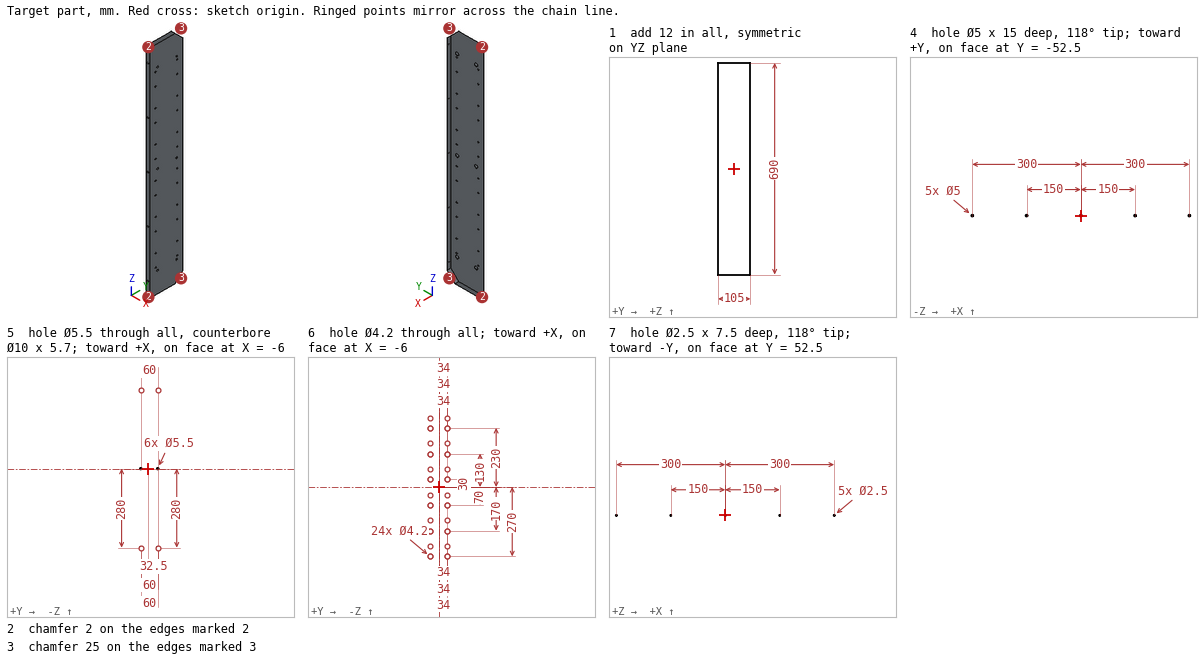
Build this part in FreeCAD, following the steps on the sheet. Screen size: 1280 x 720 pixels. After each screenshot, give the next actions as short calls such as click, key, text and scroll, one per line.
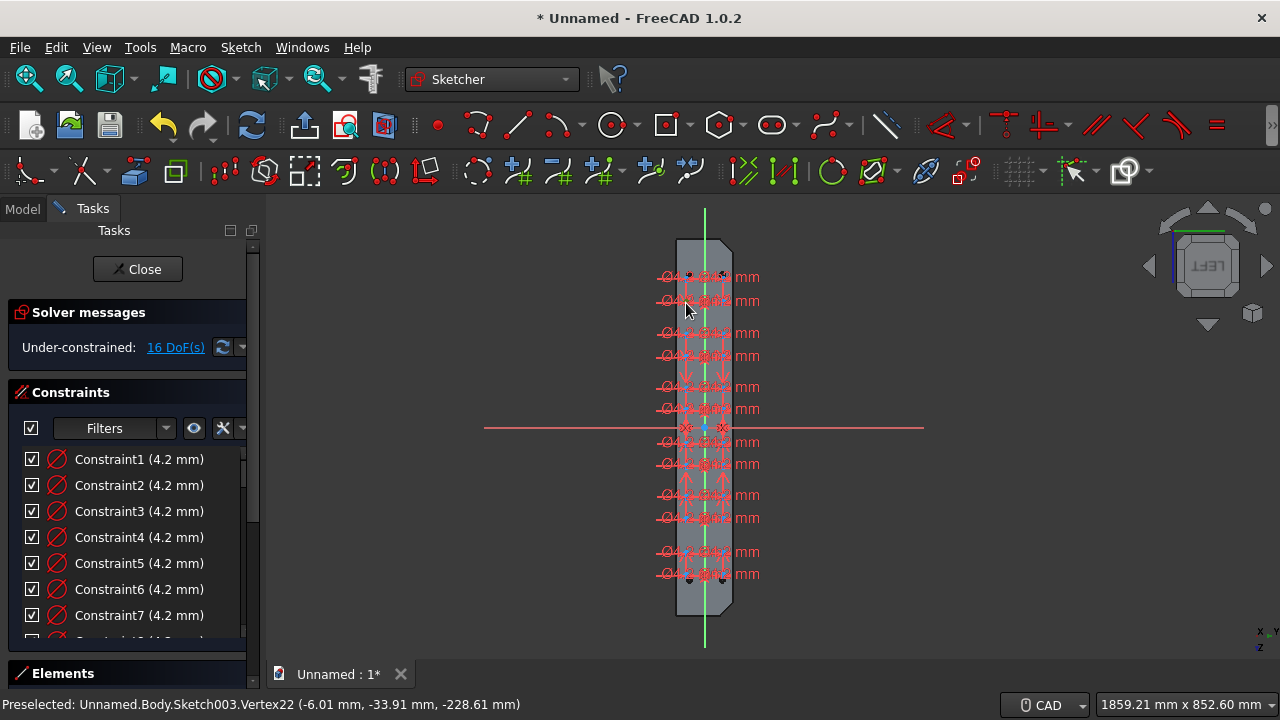
click(686, 554)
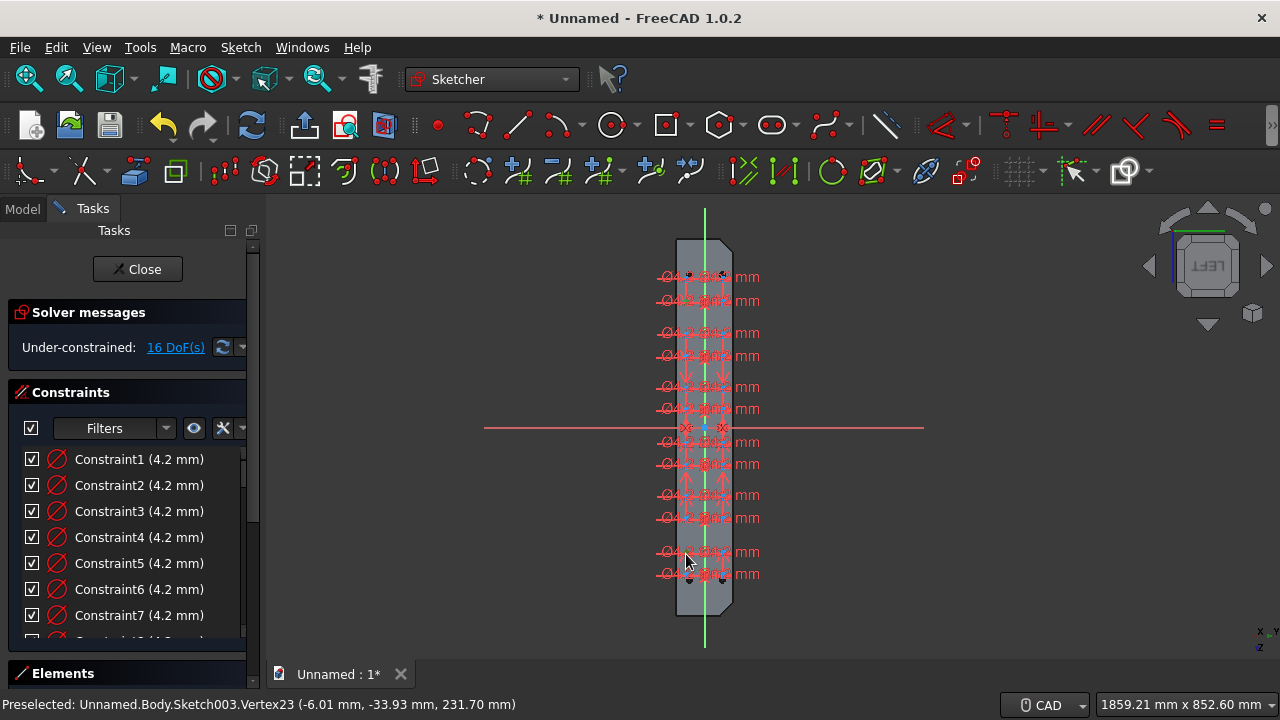
click(529, 428)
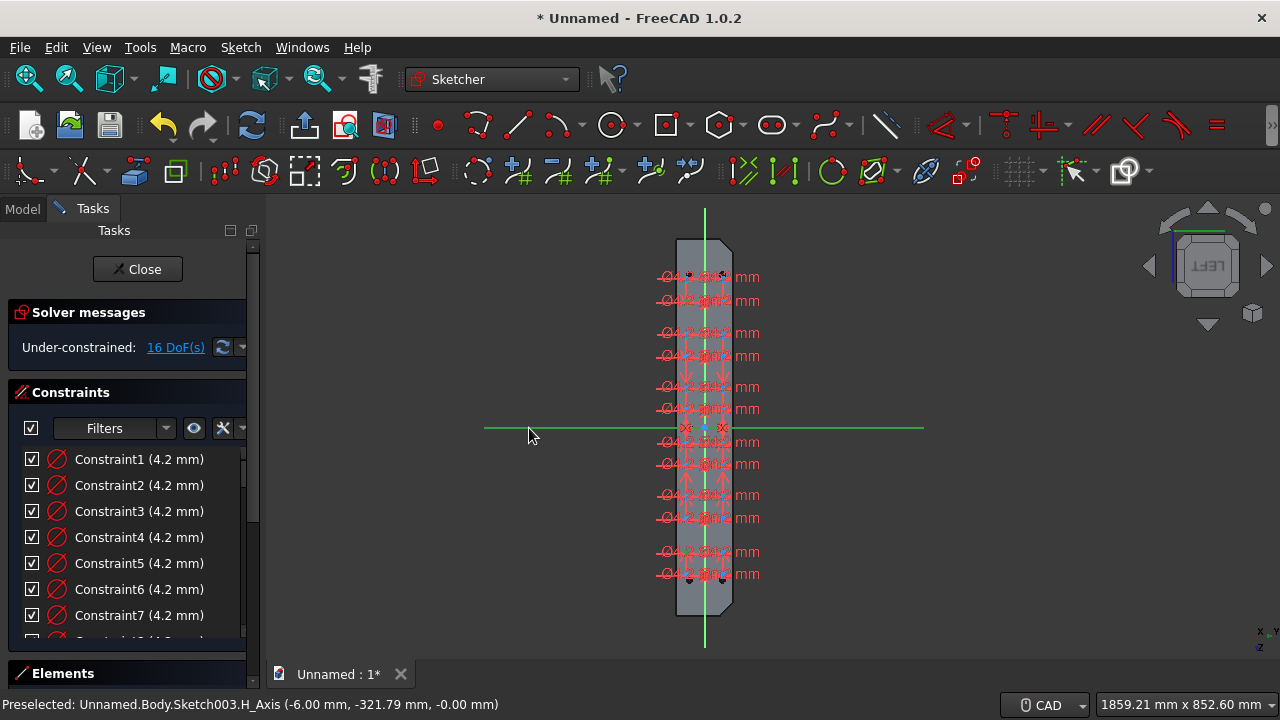
key(s)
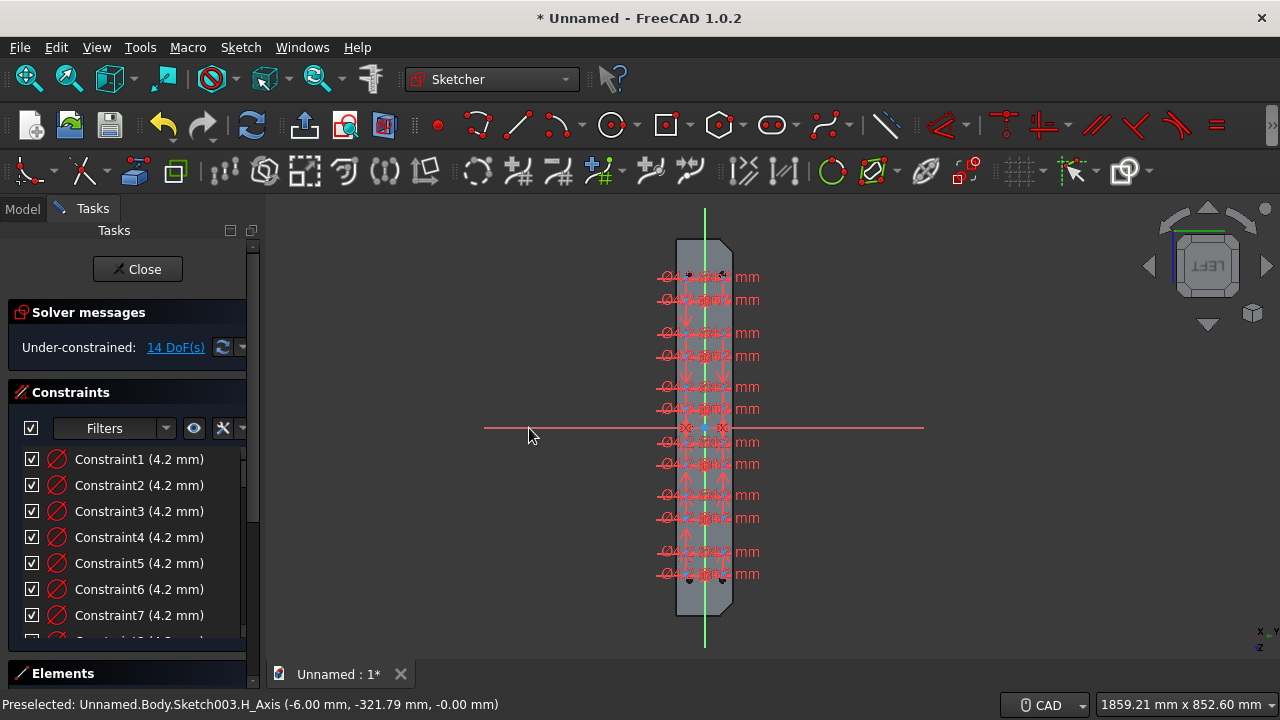
click(723, 302)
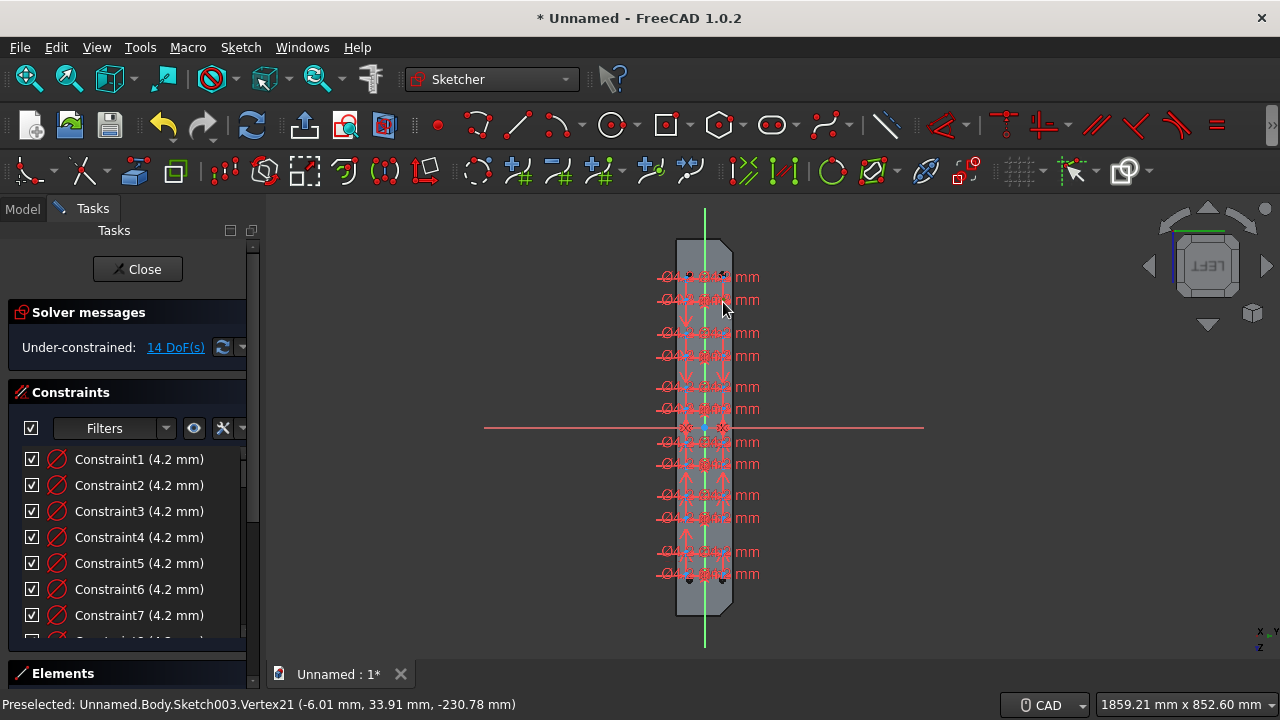
click(723, 554)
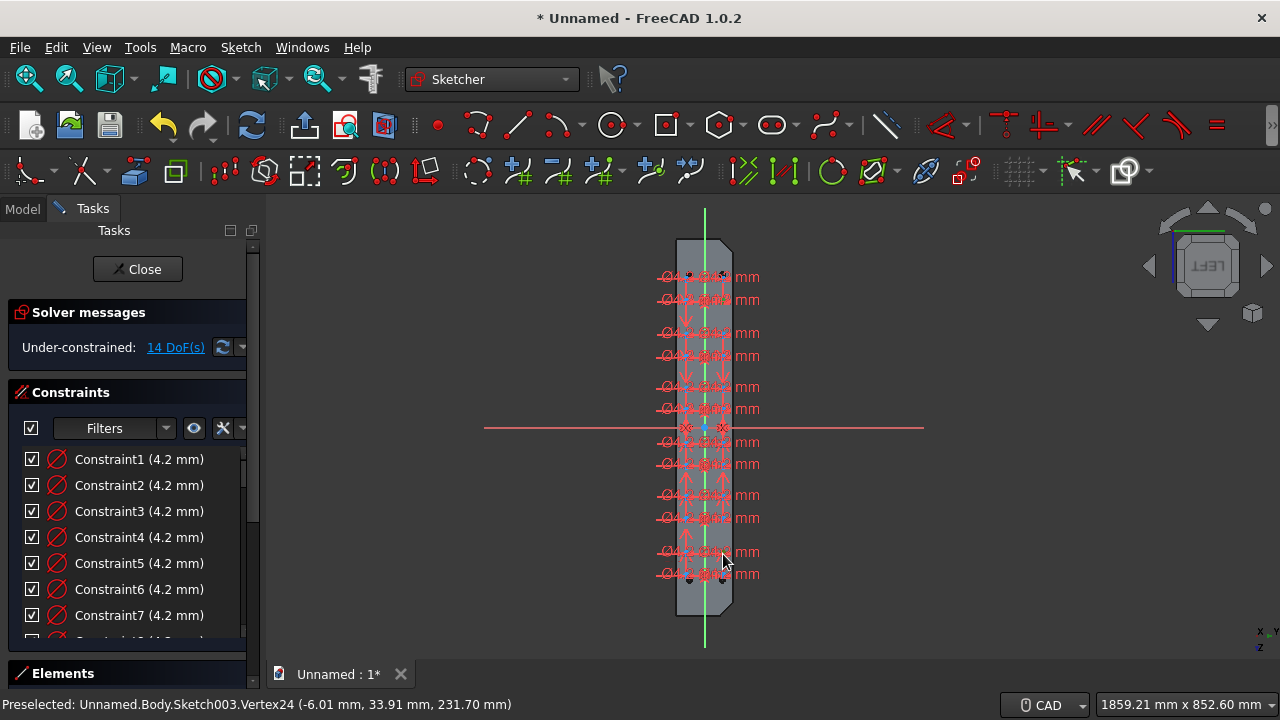
click(529, 428)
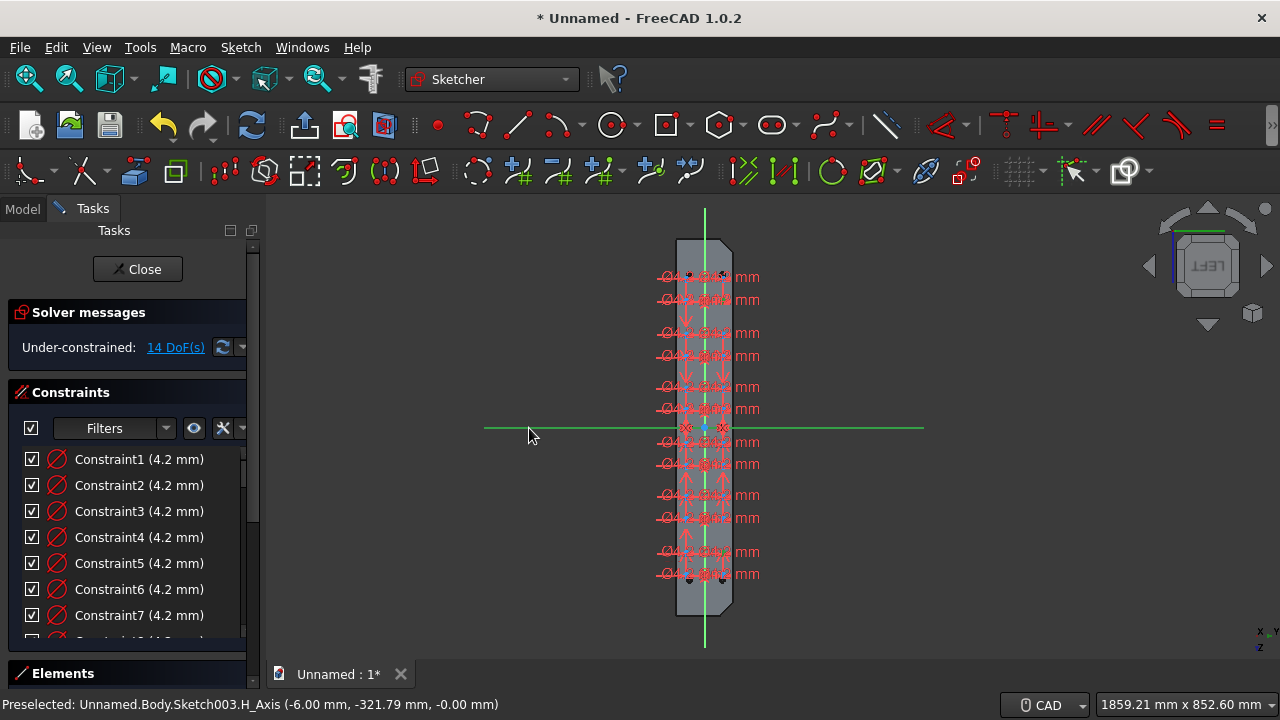
key(s)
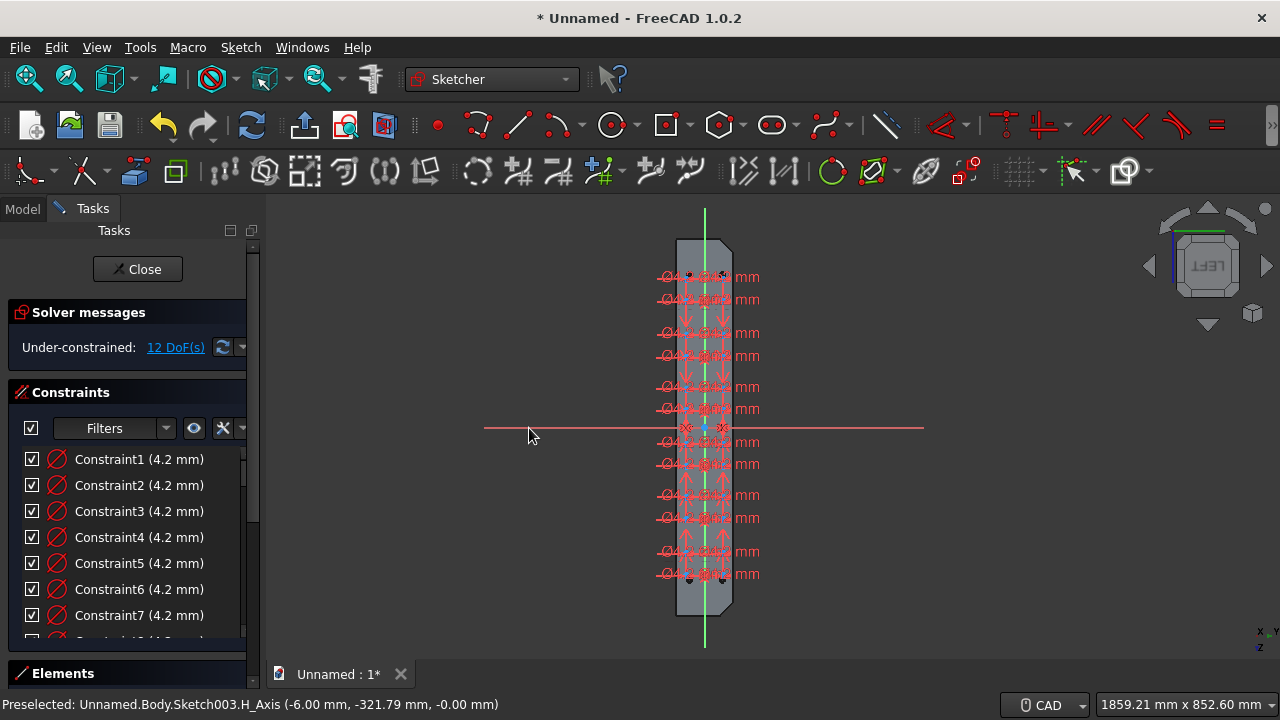
click(942, 126)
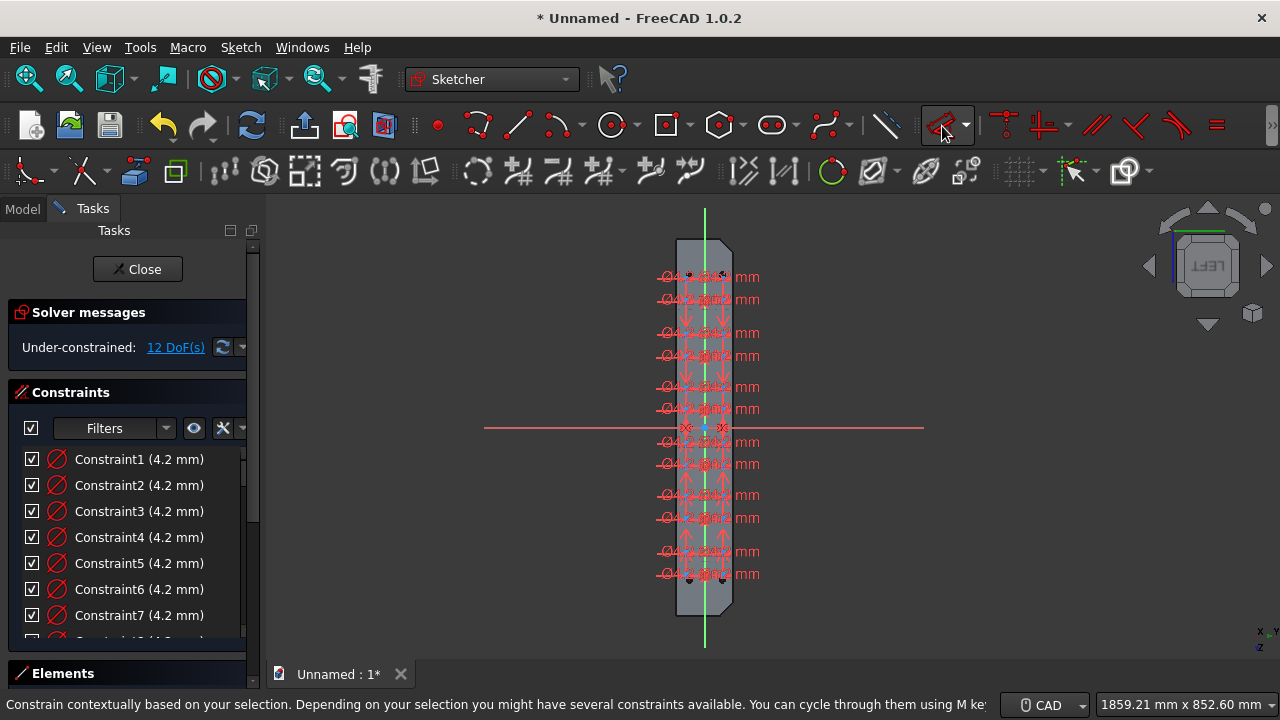
scroll(723, 576, up, 4)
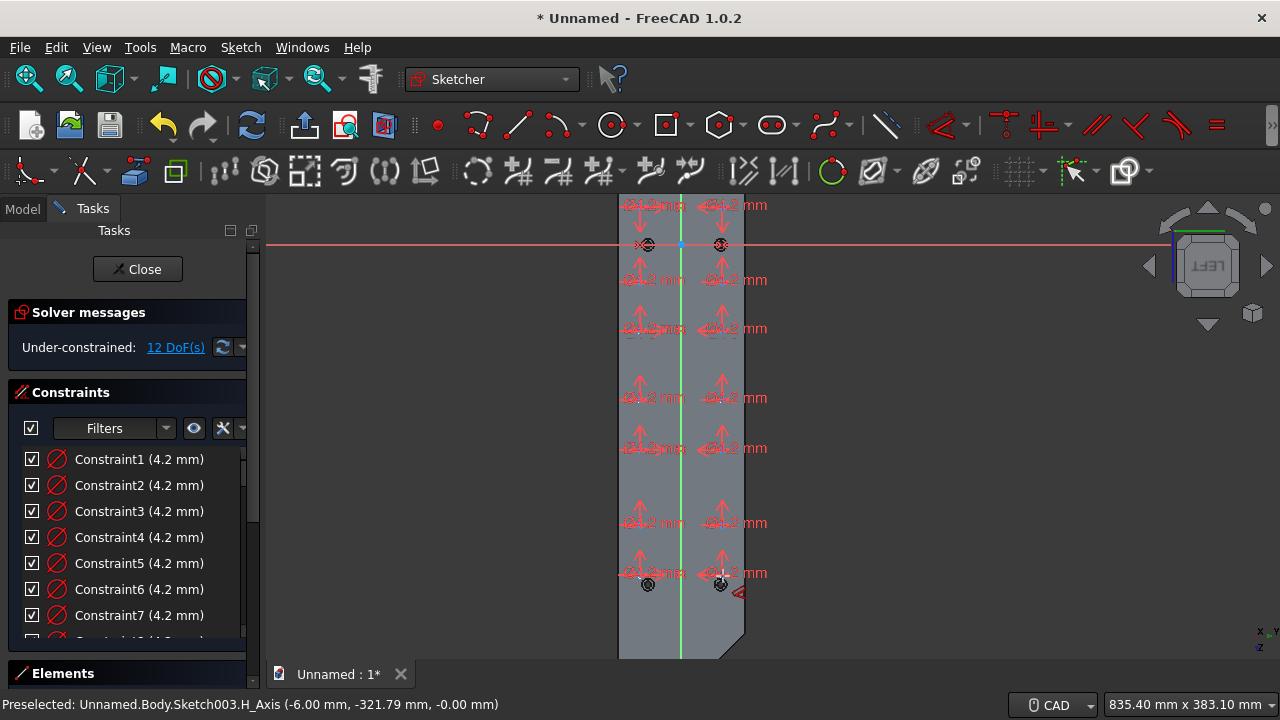
click(722, 575)
click(702, 609)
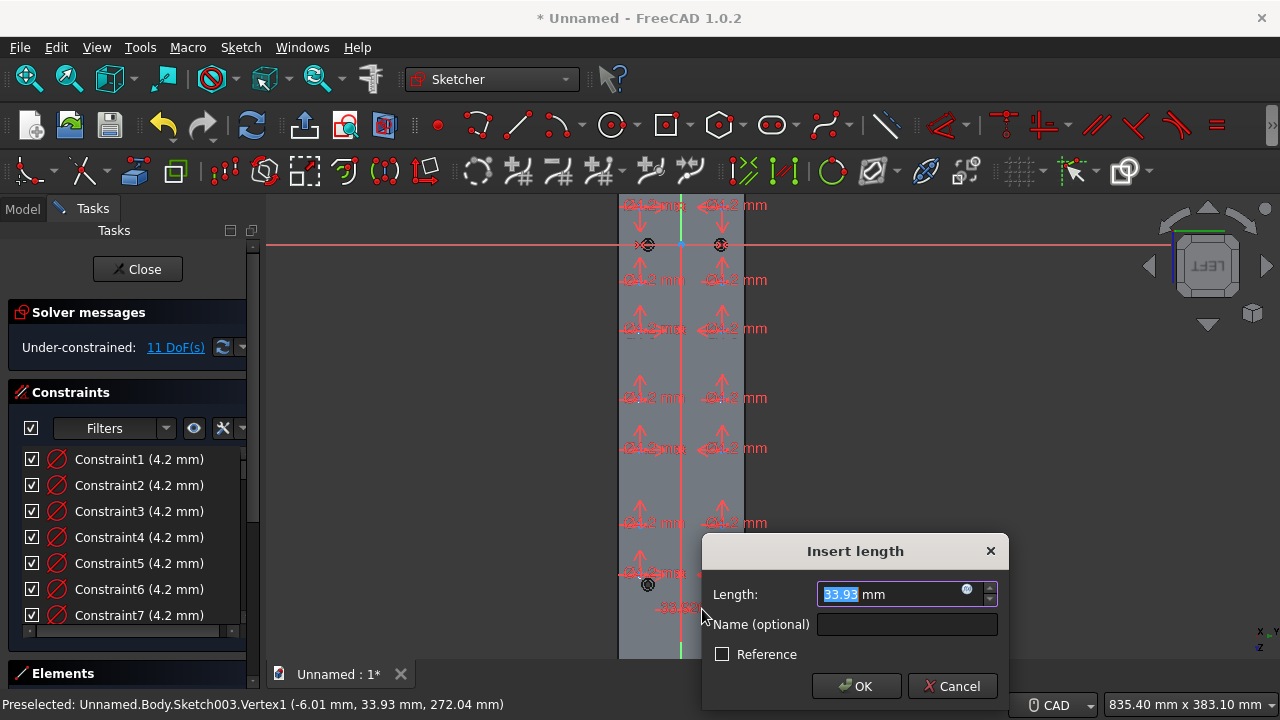
text(34)
key(Return)